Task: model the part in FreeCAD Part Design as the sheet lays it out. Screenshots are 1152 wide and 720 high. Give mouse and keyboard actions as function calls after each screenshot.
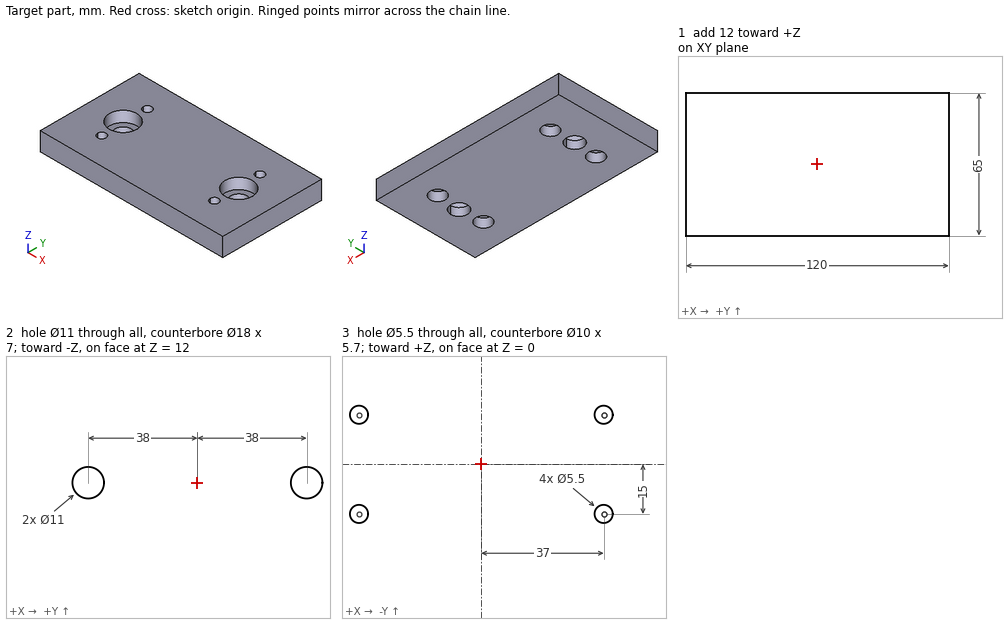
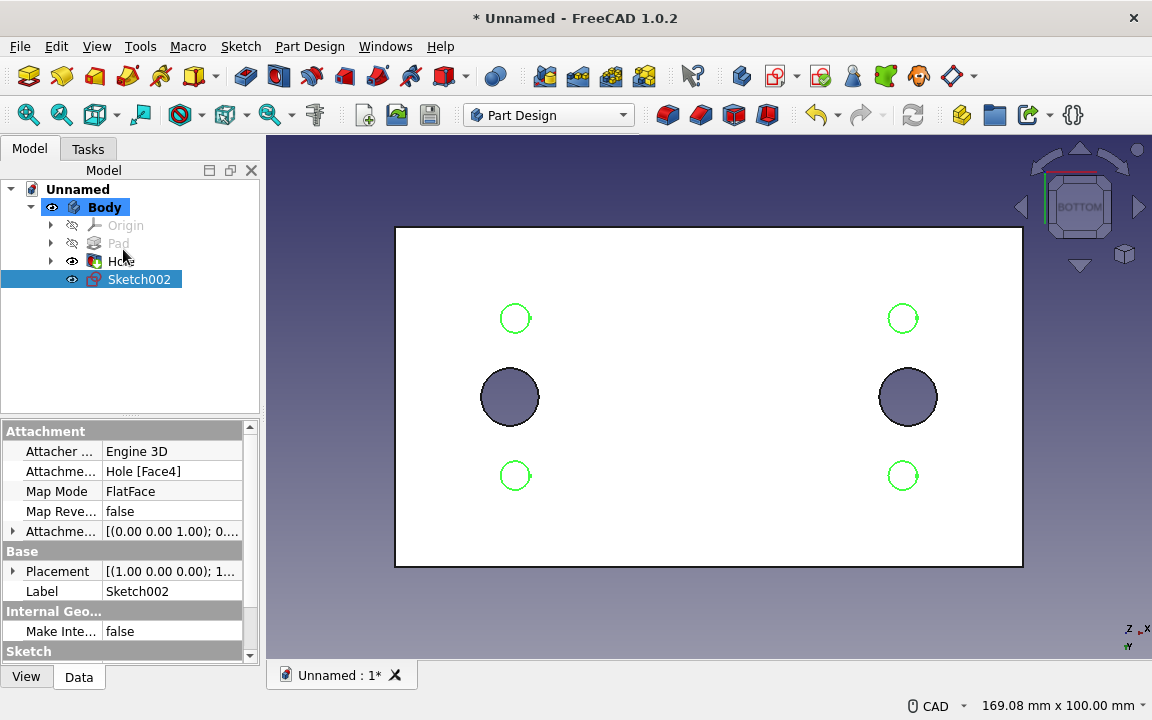
click(279, 76)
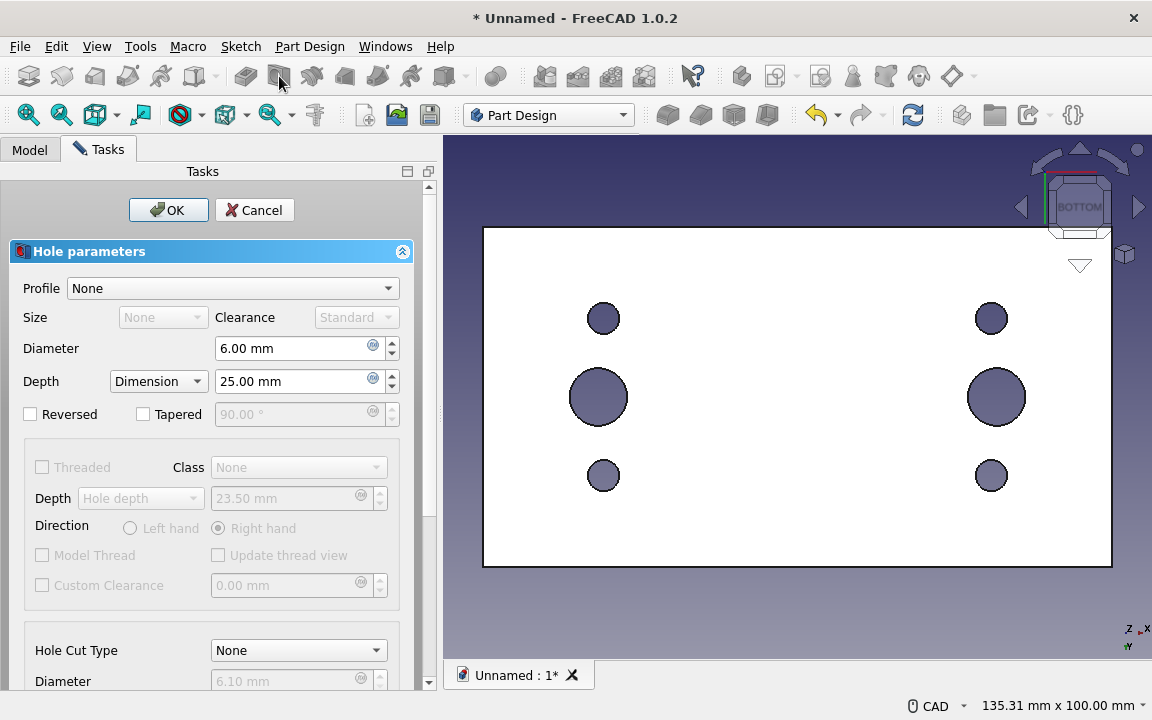
triple_click(300, 348)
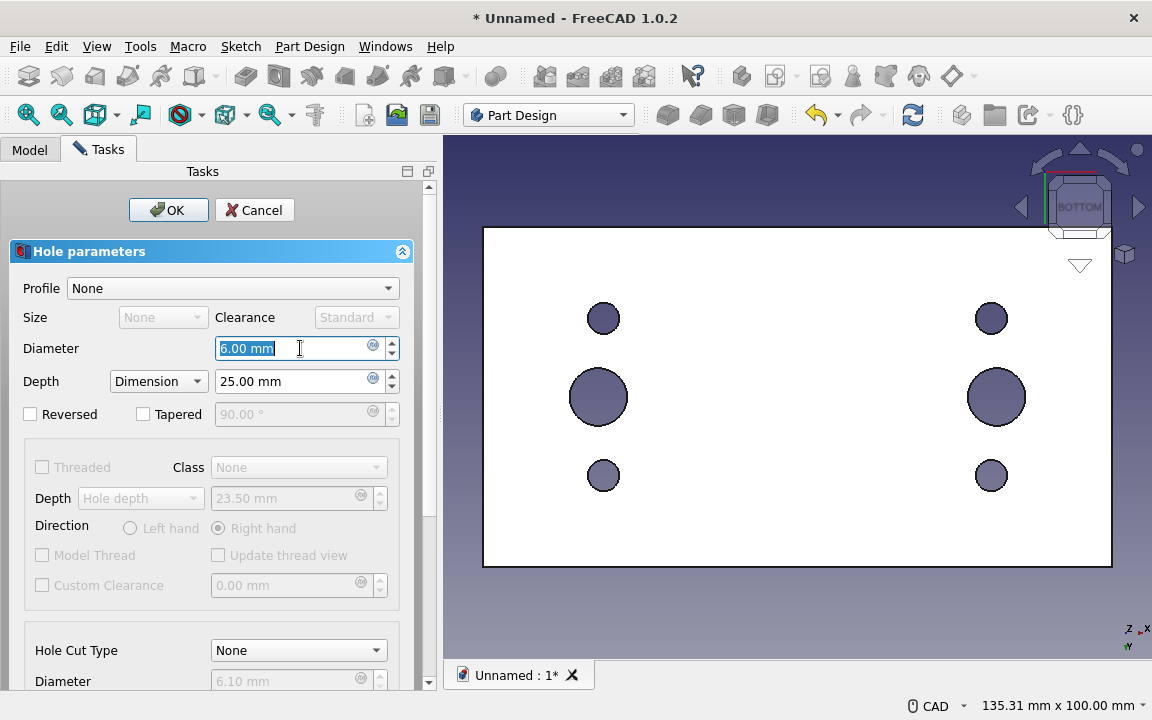
text(5.5)
key(Tab)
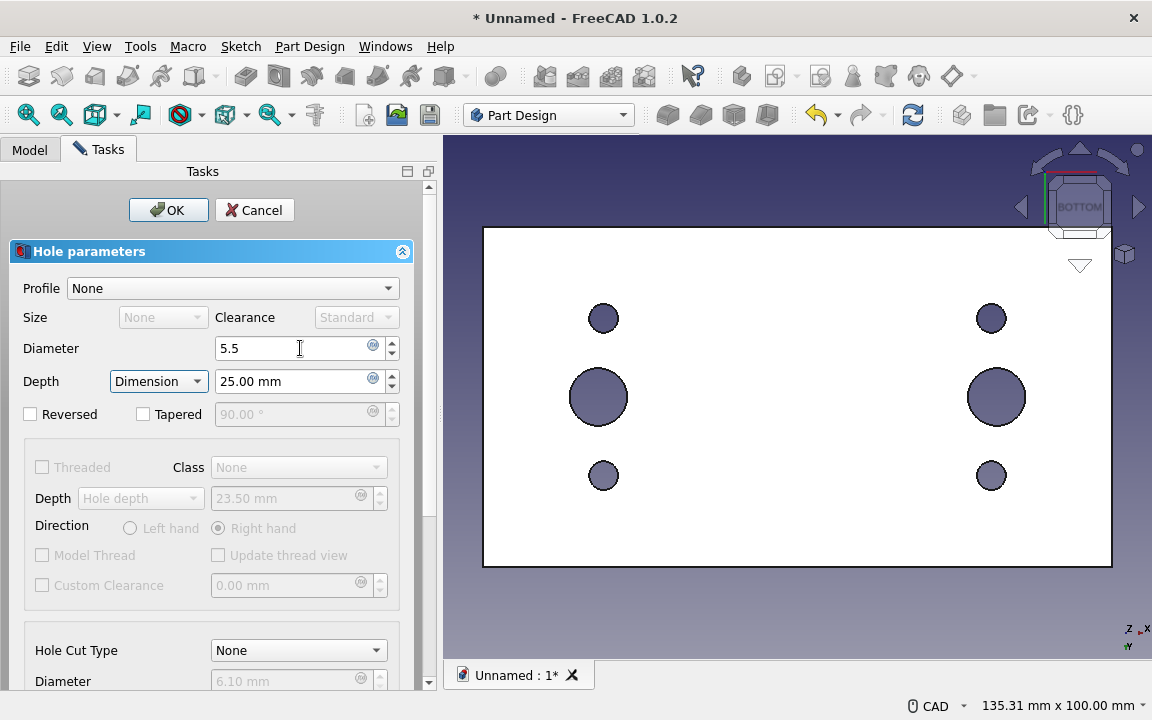
click(160, 382)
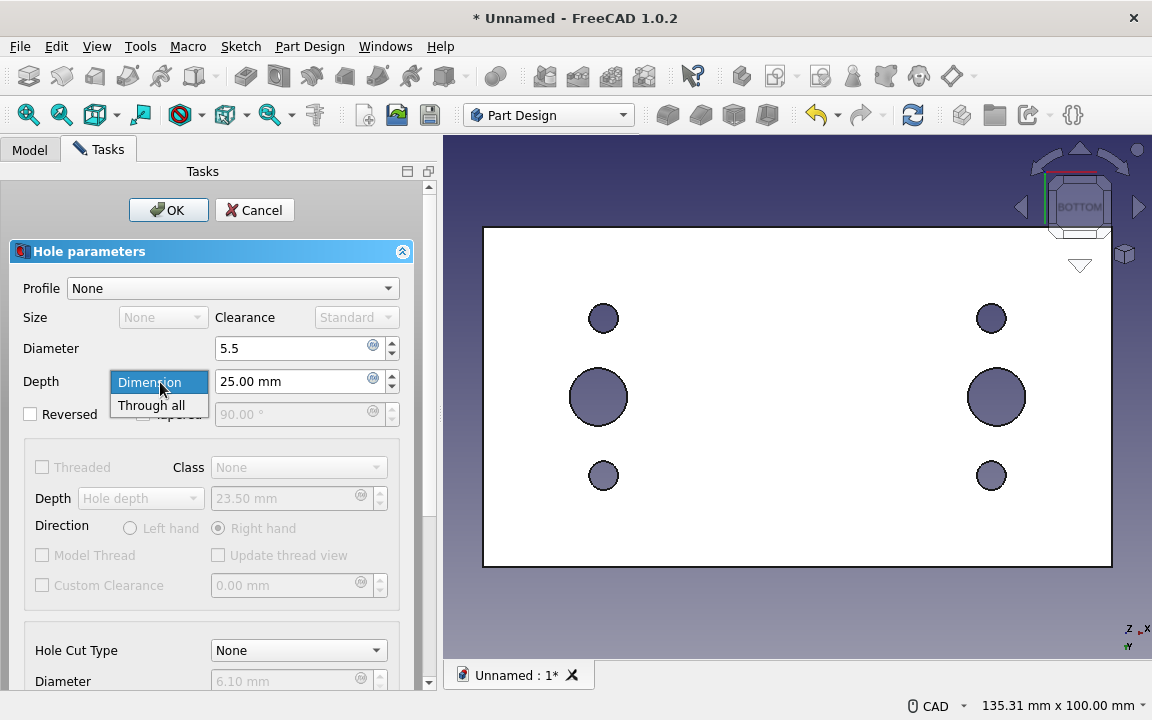
click(158, 406)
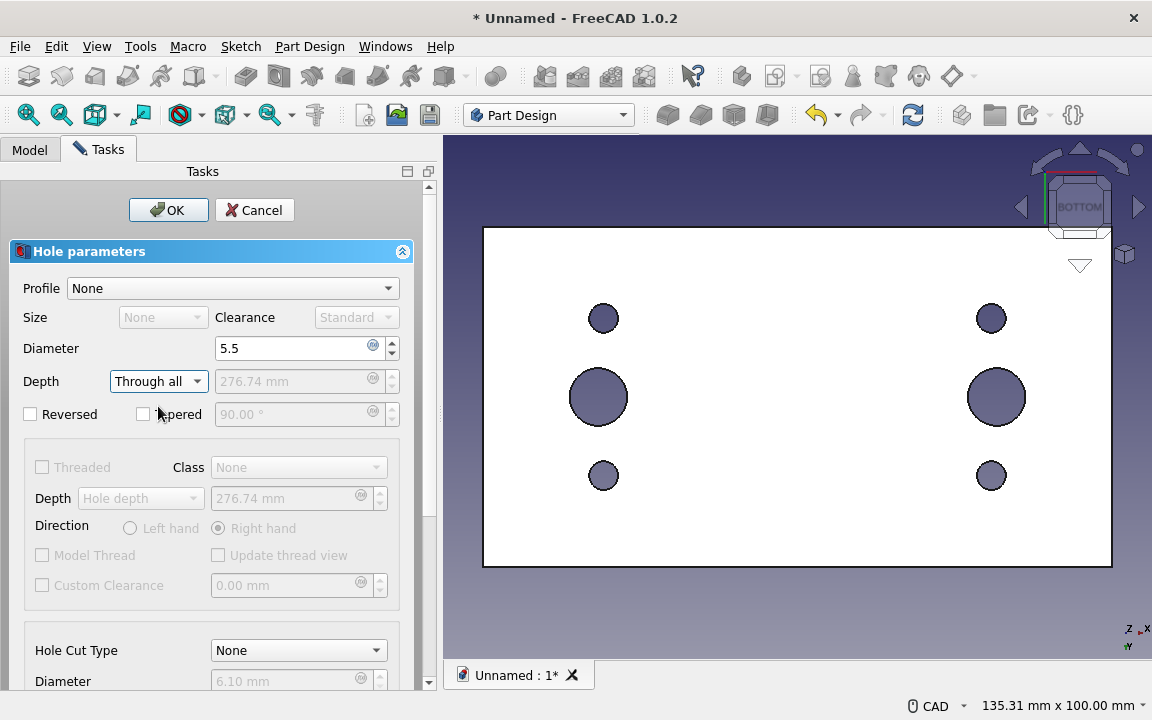
click(300, 650)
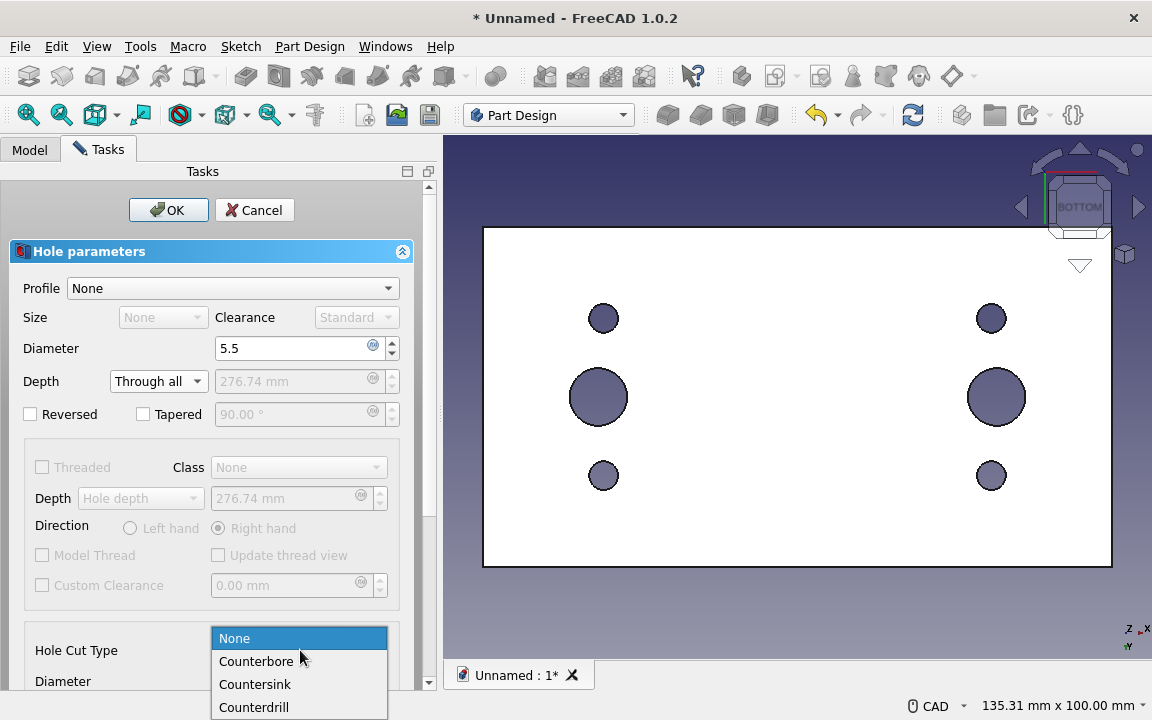
click(298, 662)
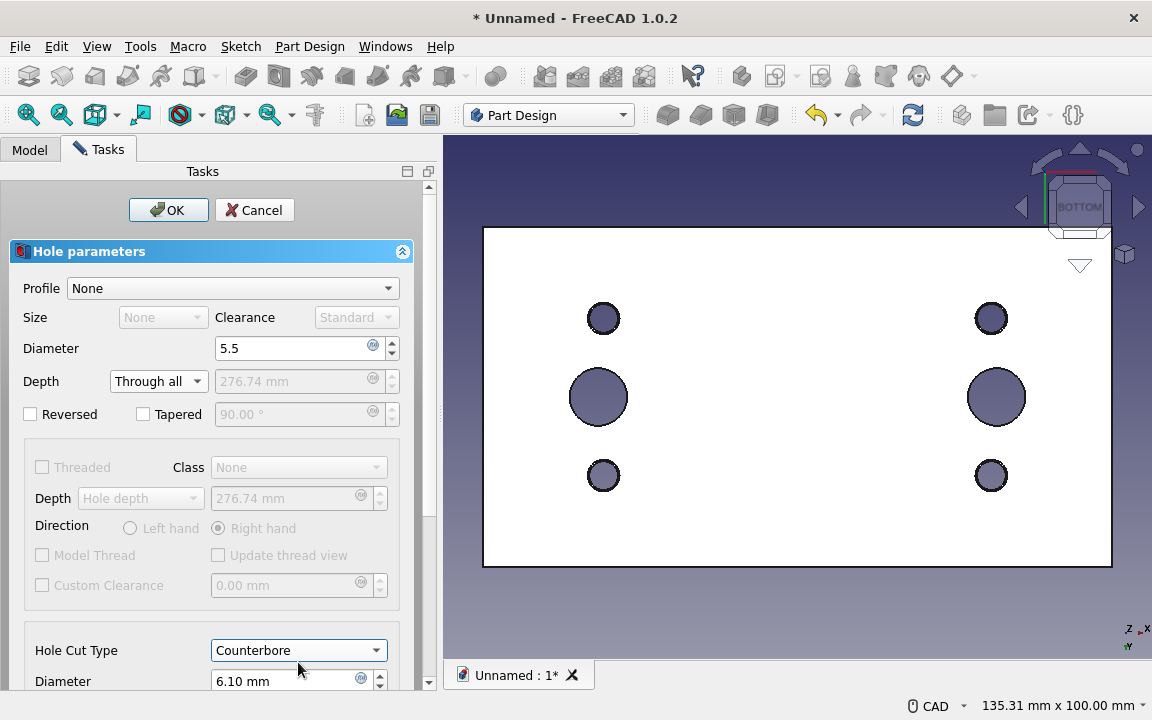
scroll(429, 436, down, 2)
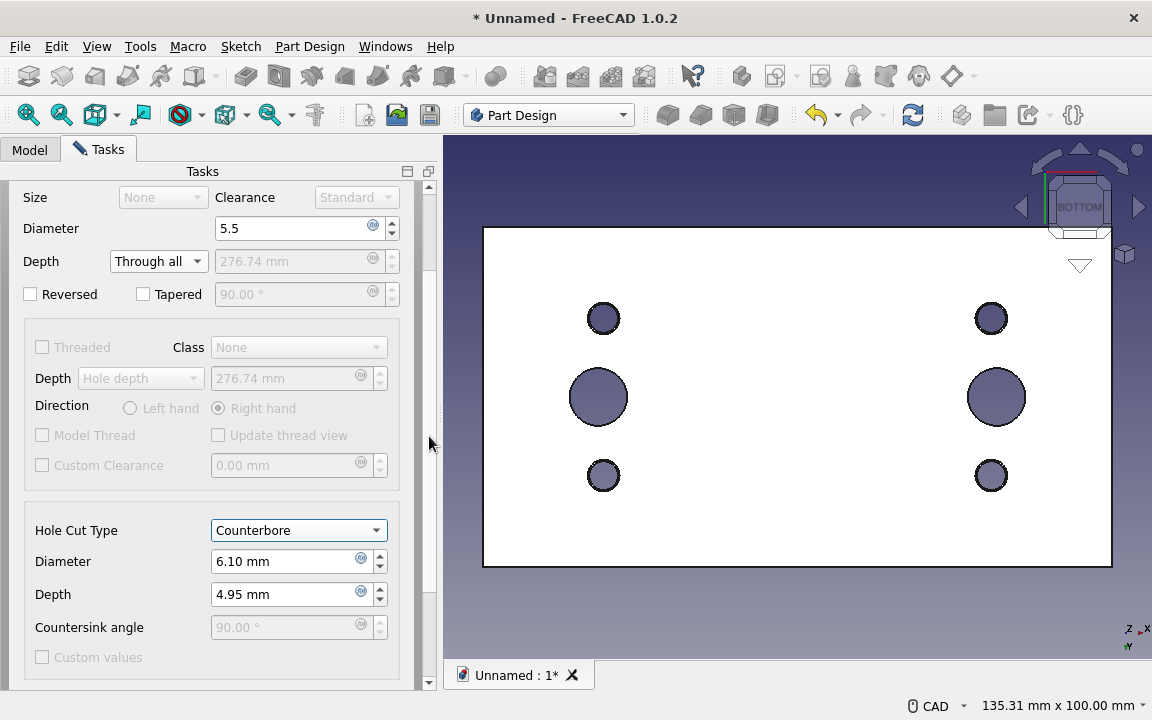
triple_click(292, 562)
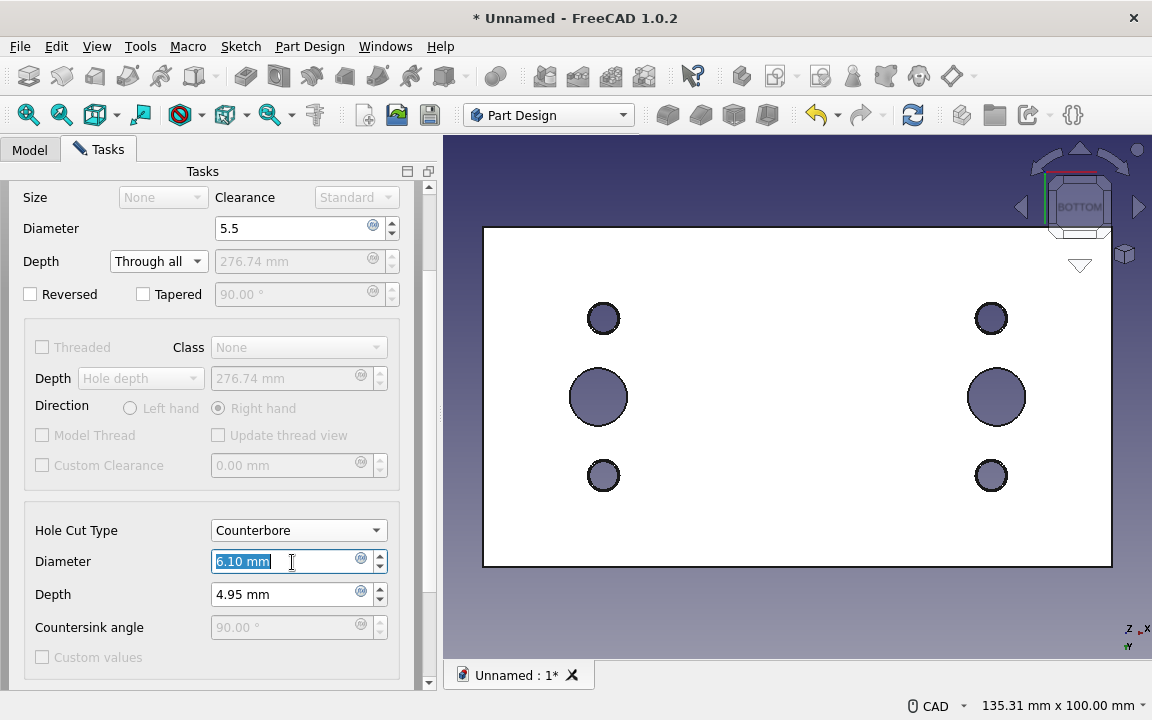
text(10)
key(Tab)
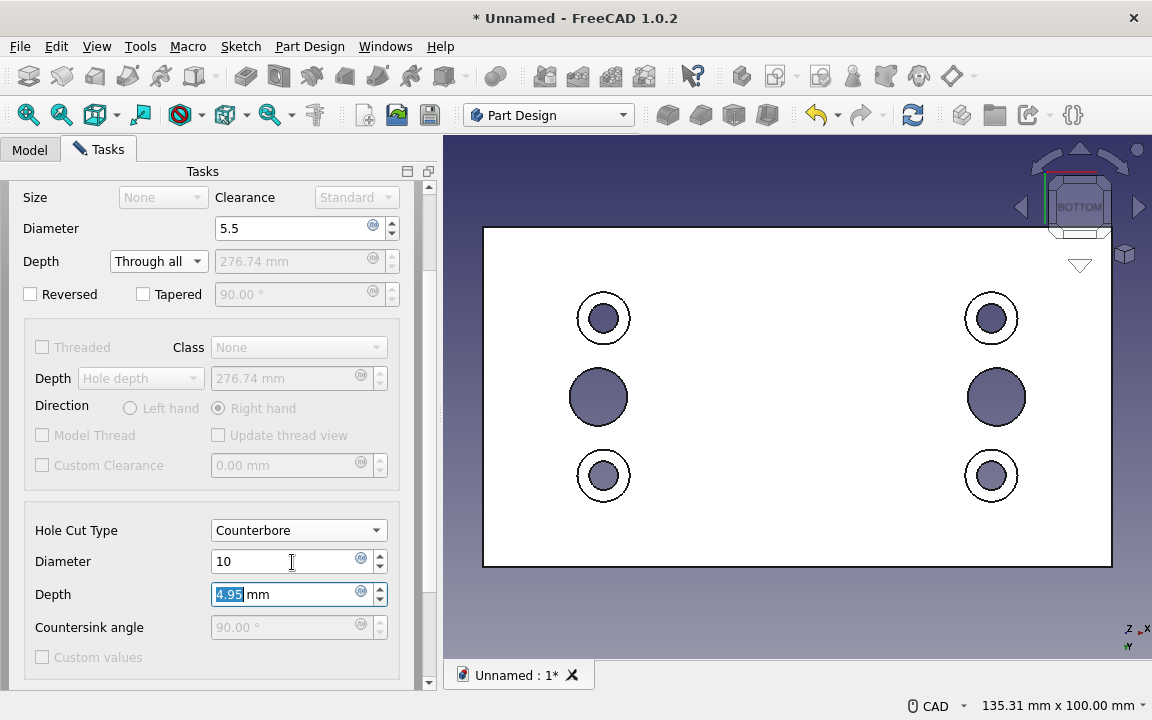
text(5.7)
key(Tab)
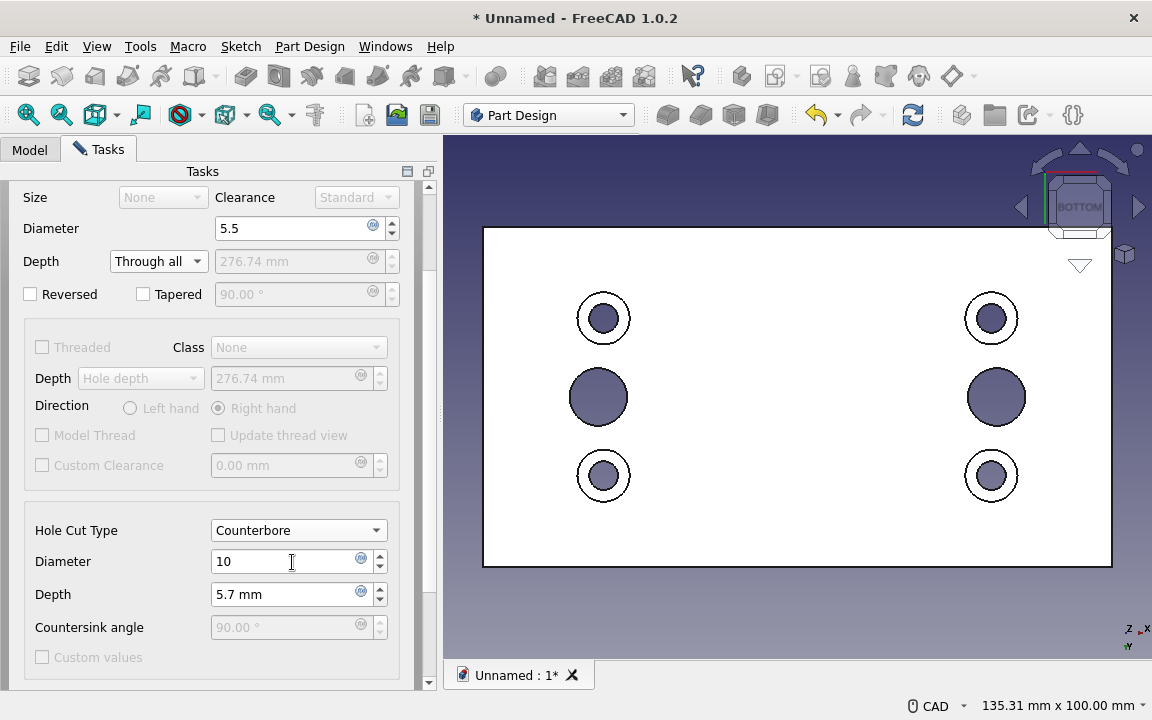
scroll(429, 436, up, 3)